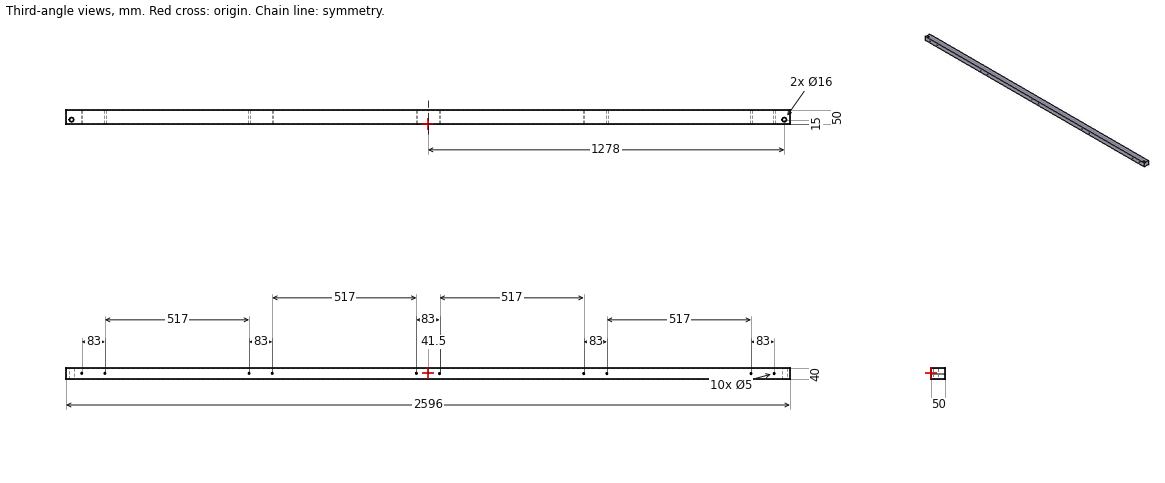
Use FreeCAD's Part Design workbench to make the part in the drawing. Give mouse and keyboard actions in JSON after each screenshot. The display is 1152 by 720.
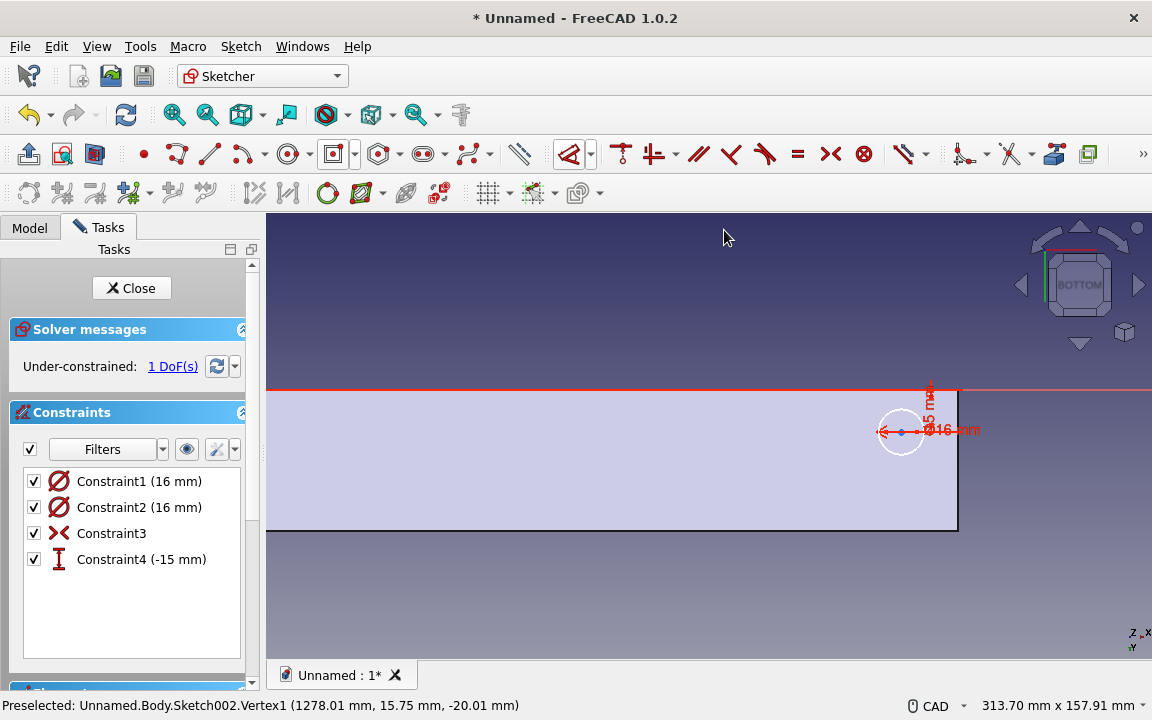
{"action": "scroll", "coordinate": [909, 437], "scroll_direction": "down", "scroll_amount": 13}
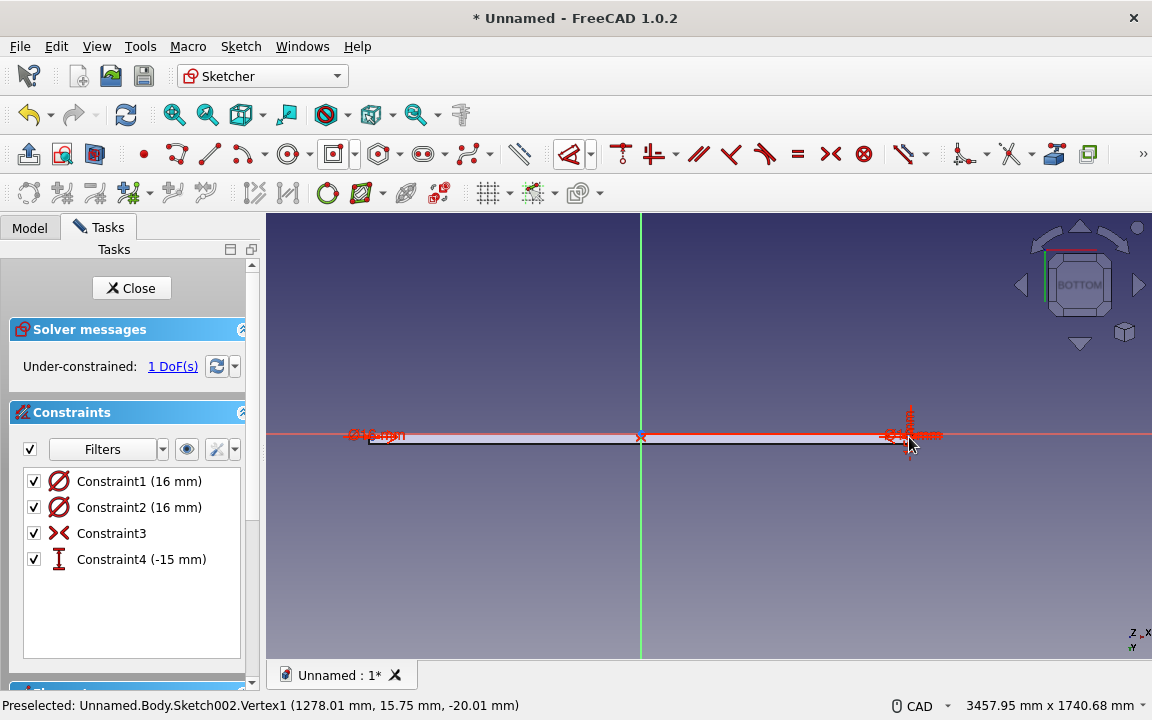
{"action": "left_click", "coordinate": [909, 437]}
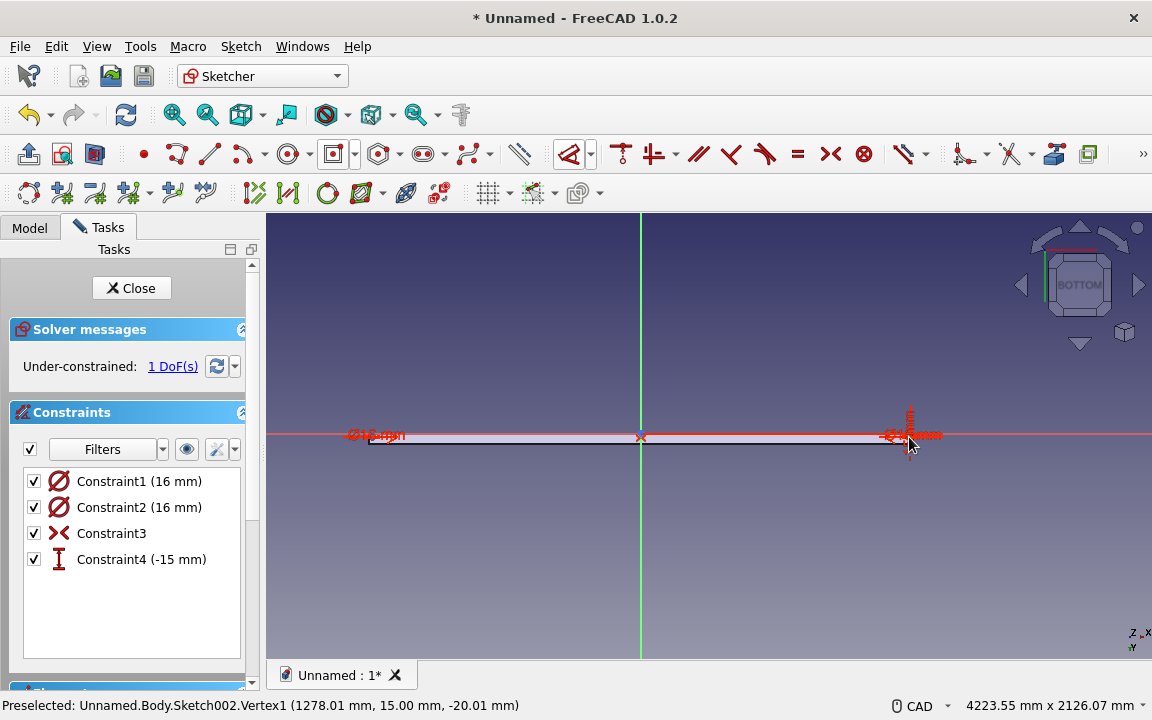
{"action": "left_click", "coordinate": [590, 154]}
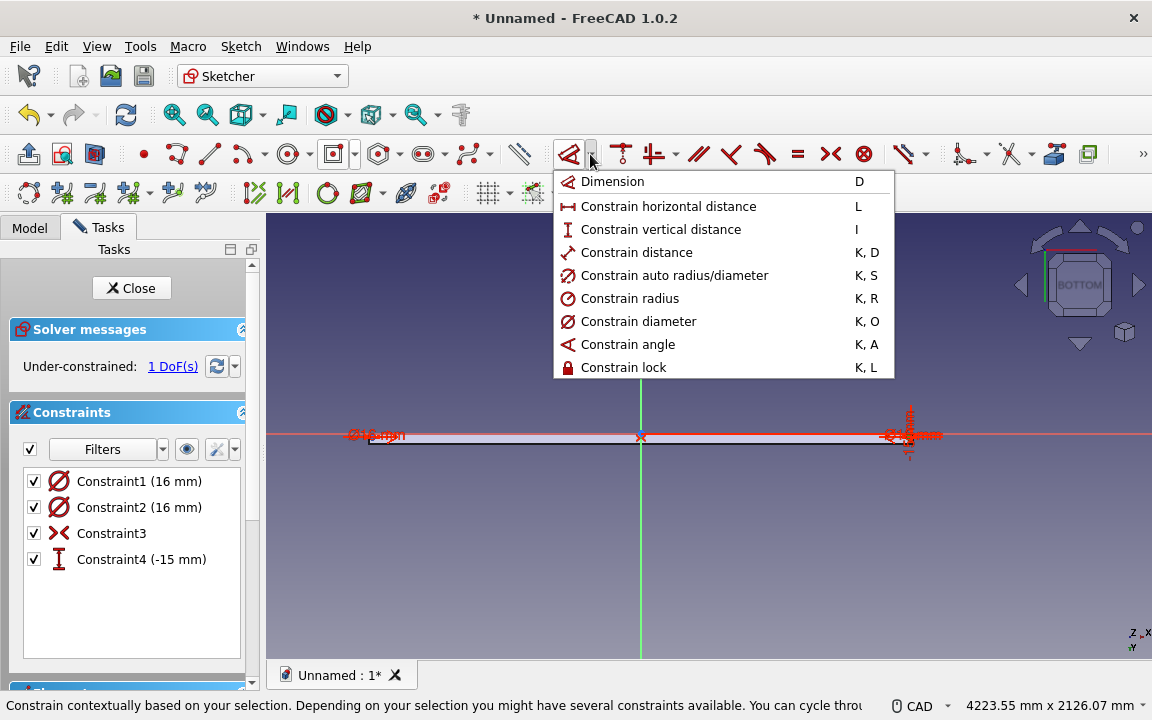
{"action": "left_click", "coordinate": [724, 206]}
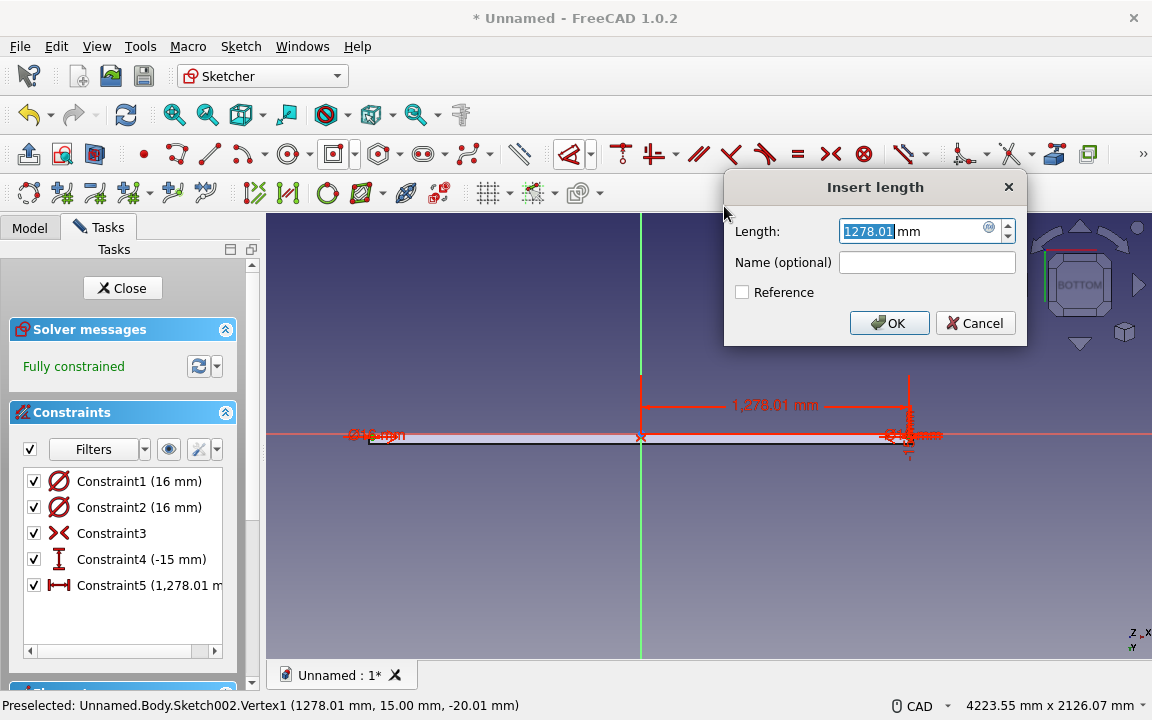
{"action": "type", "text": "1278"}
{"action": "key", "text": "Return"}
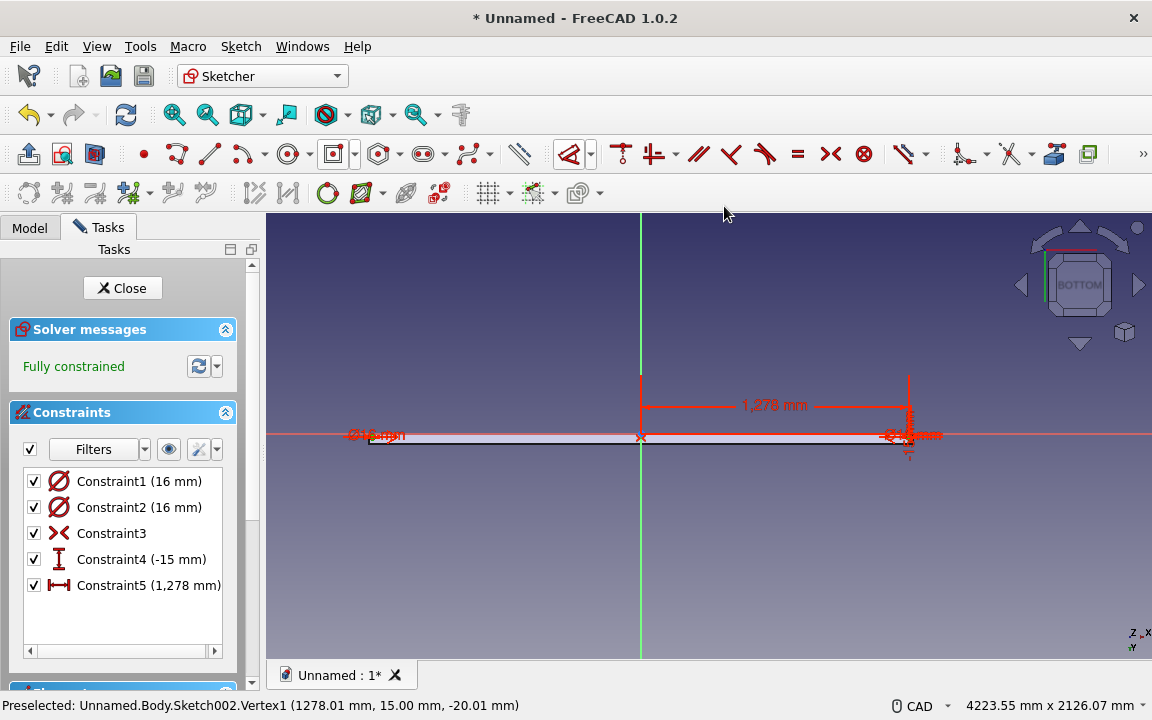
{"action": "left_click", "coordinate": [123, 288]}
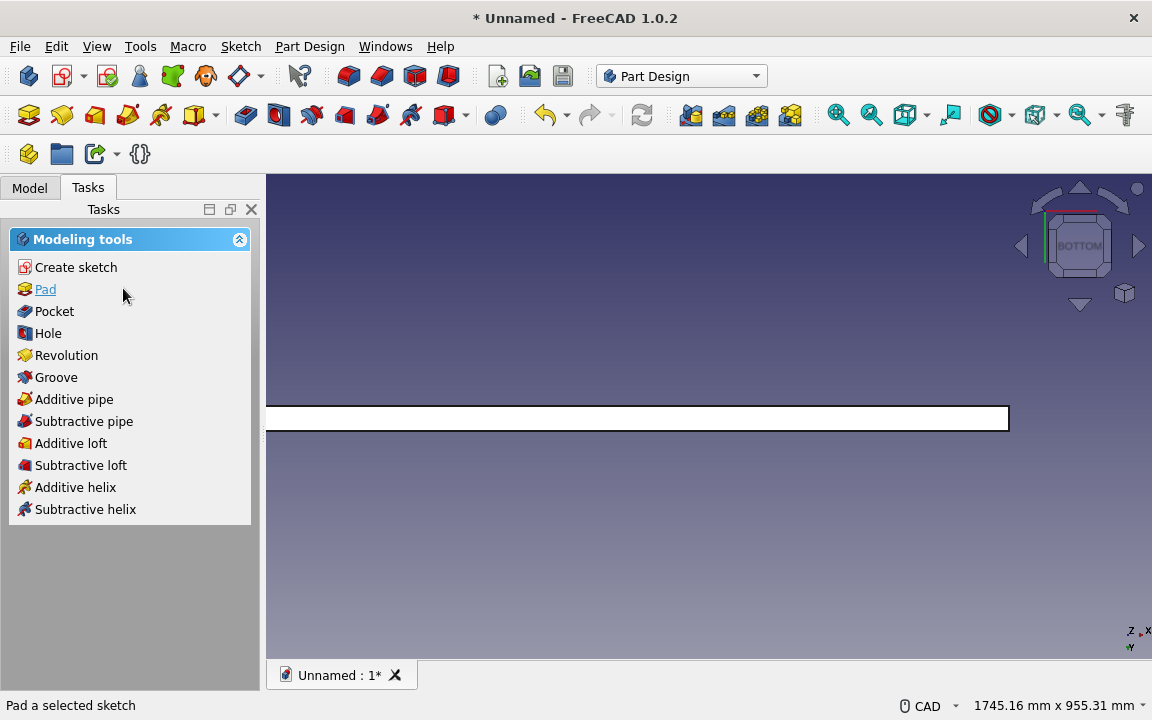
{"action": "left_click", "coordinate": [246, 116]}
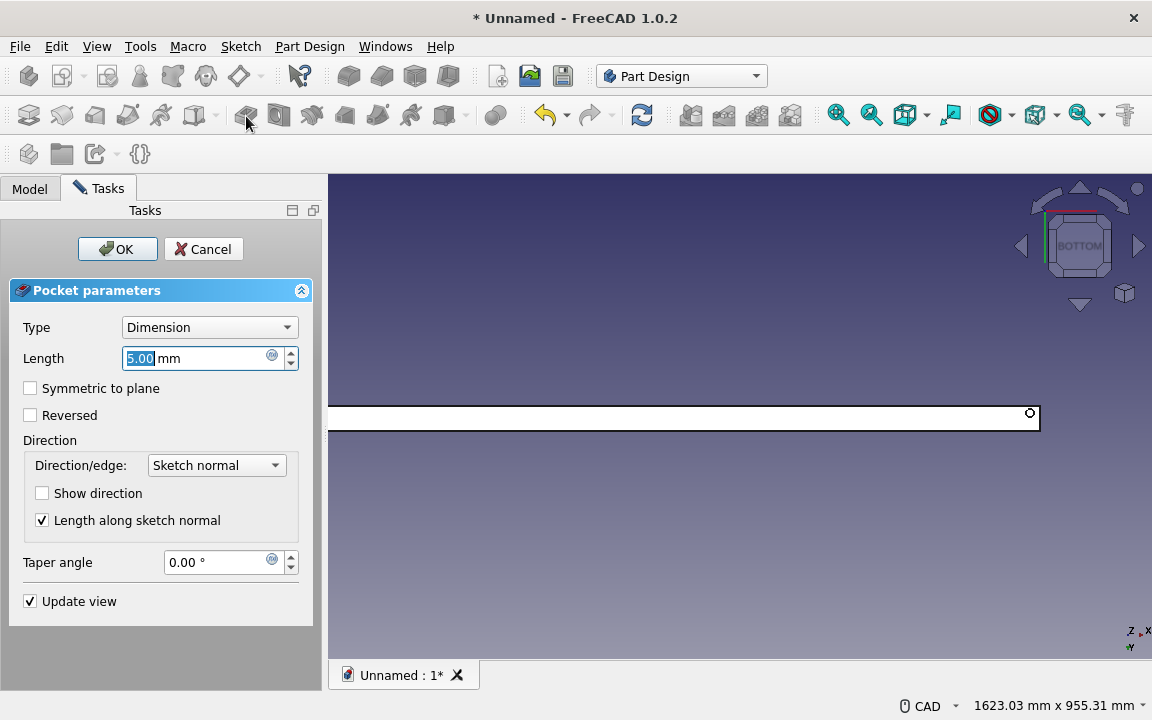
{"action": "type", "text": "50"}
{"action": "key", "text": "Tab"}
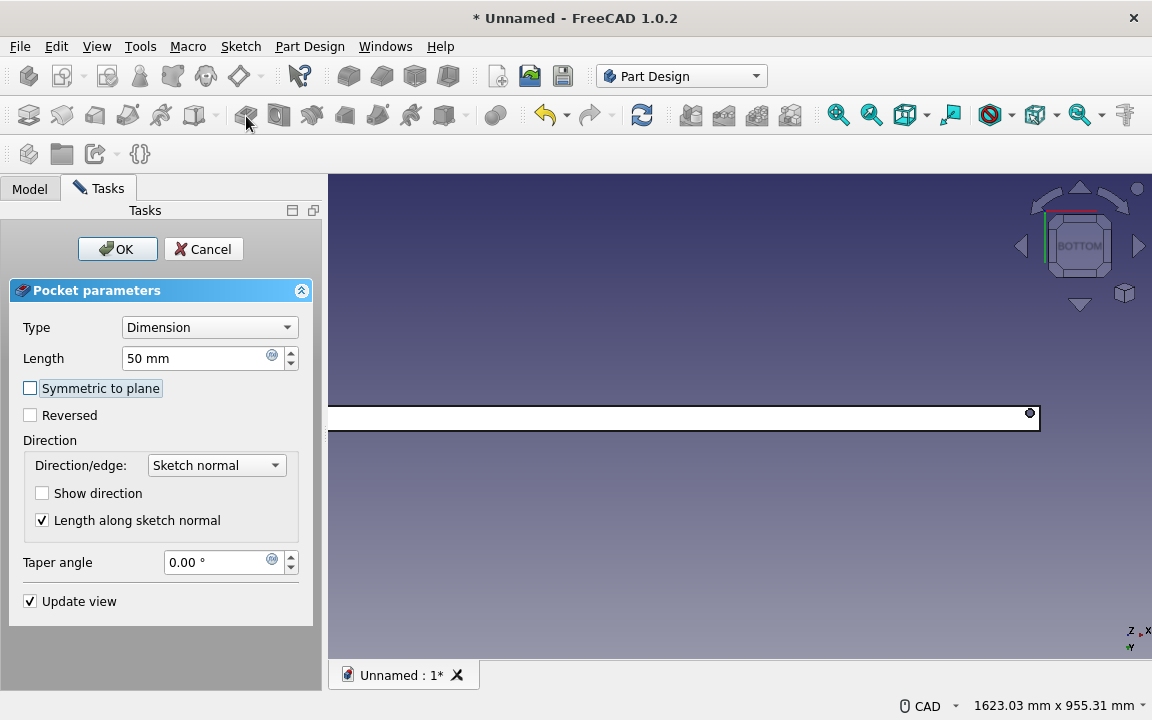
{"action": "left_click", "coordinate": [118, 249]}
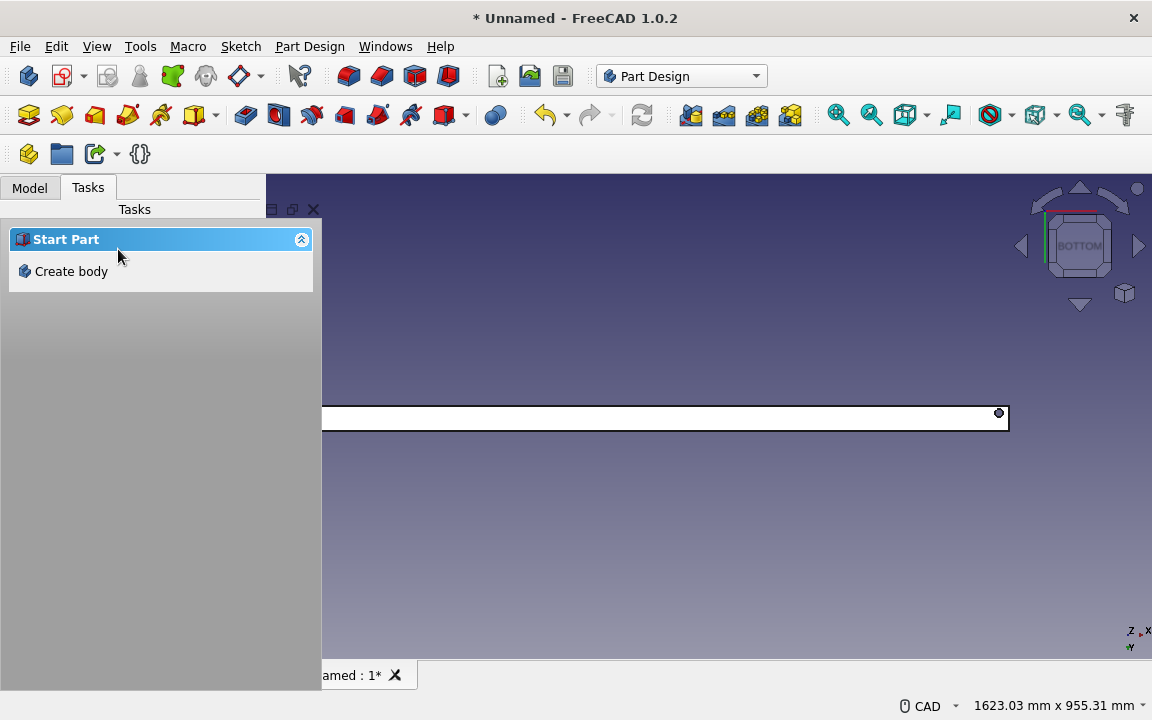
{"action": "key", "text": "0"}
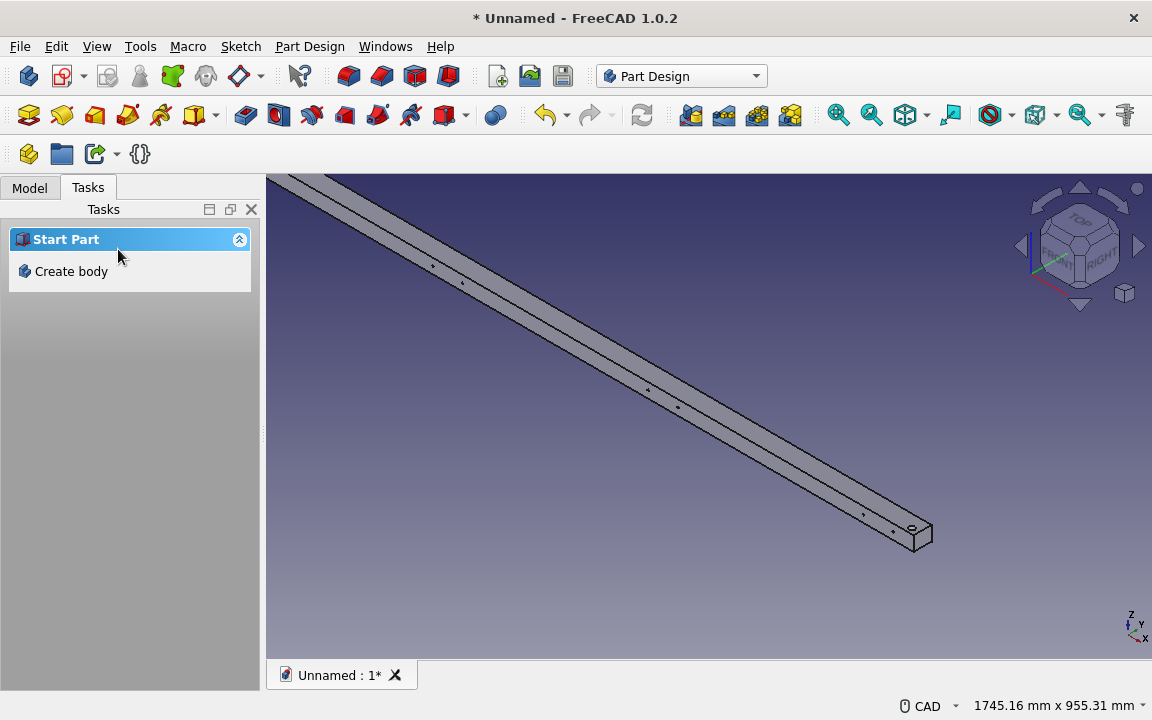
{"action": "left_click", "coordinate": [839, 116]}